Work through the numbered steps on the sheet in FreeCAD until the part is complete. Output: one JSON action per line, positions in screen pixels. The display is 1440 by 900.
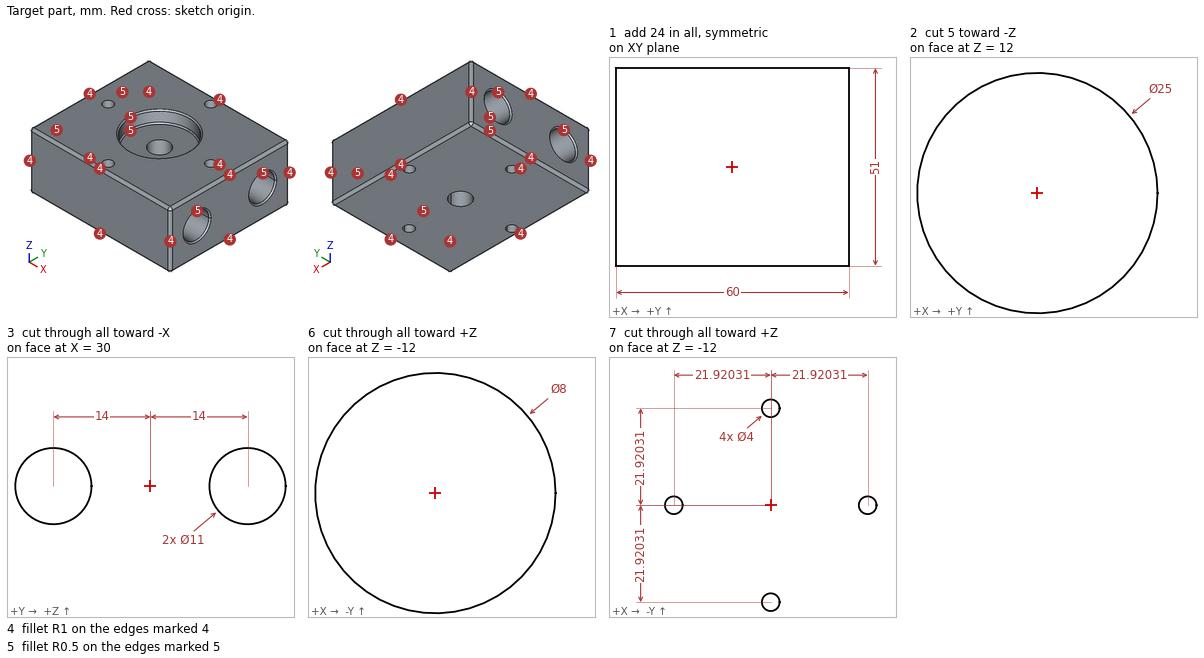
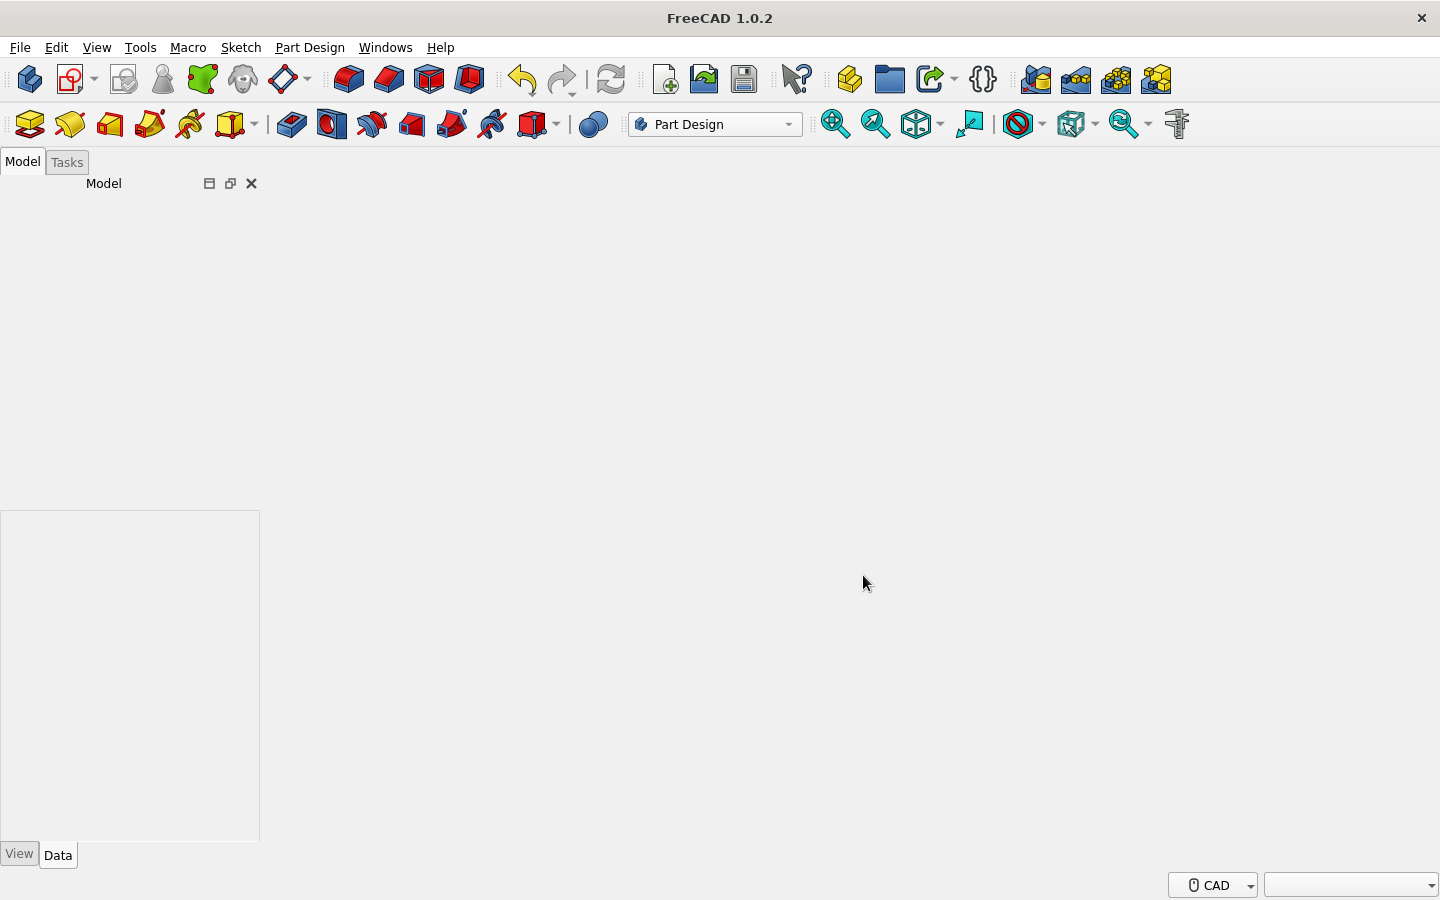
{"action": "left_click", "coordinate": [664, 80]}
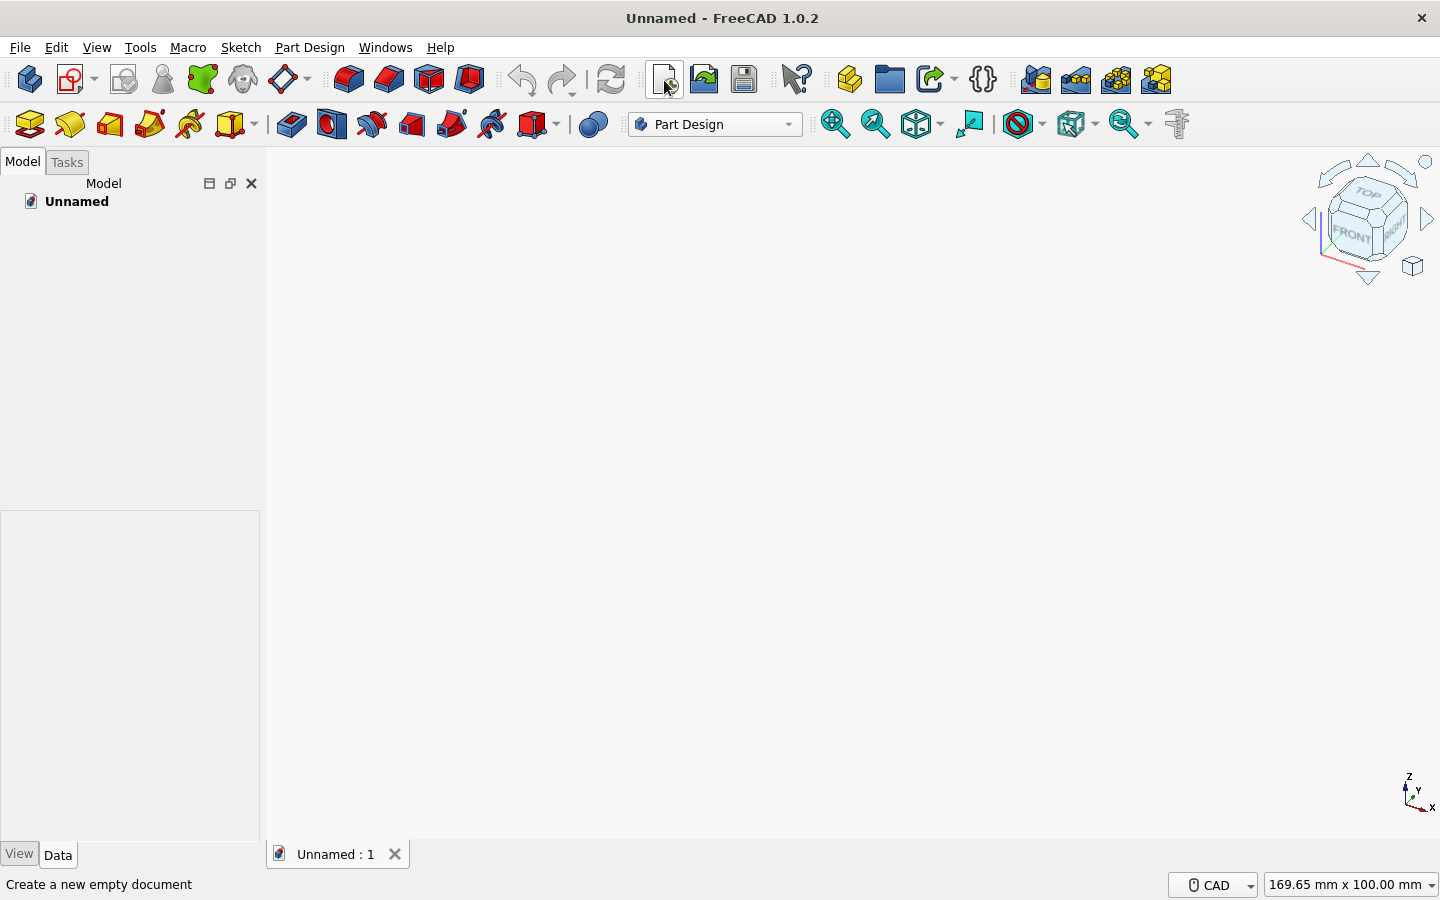
{"action": "left_click", "coordinate": [70, 80]}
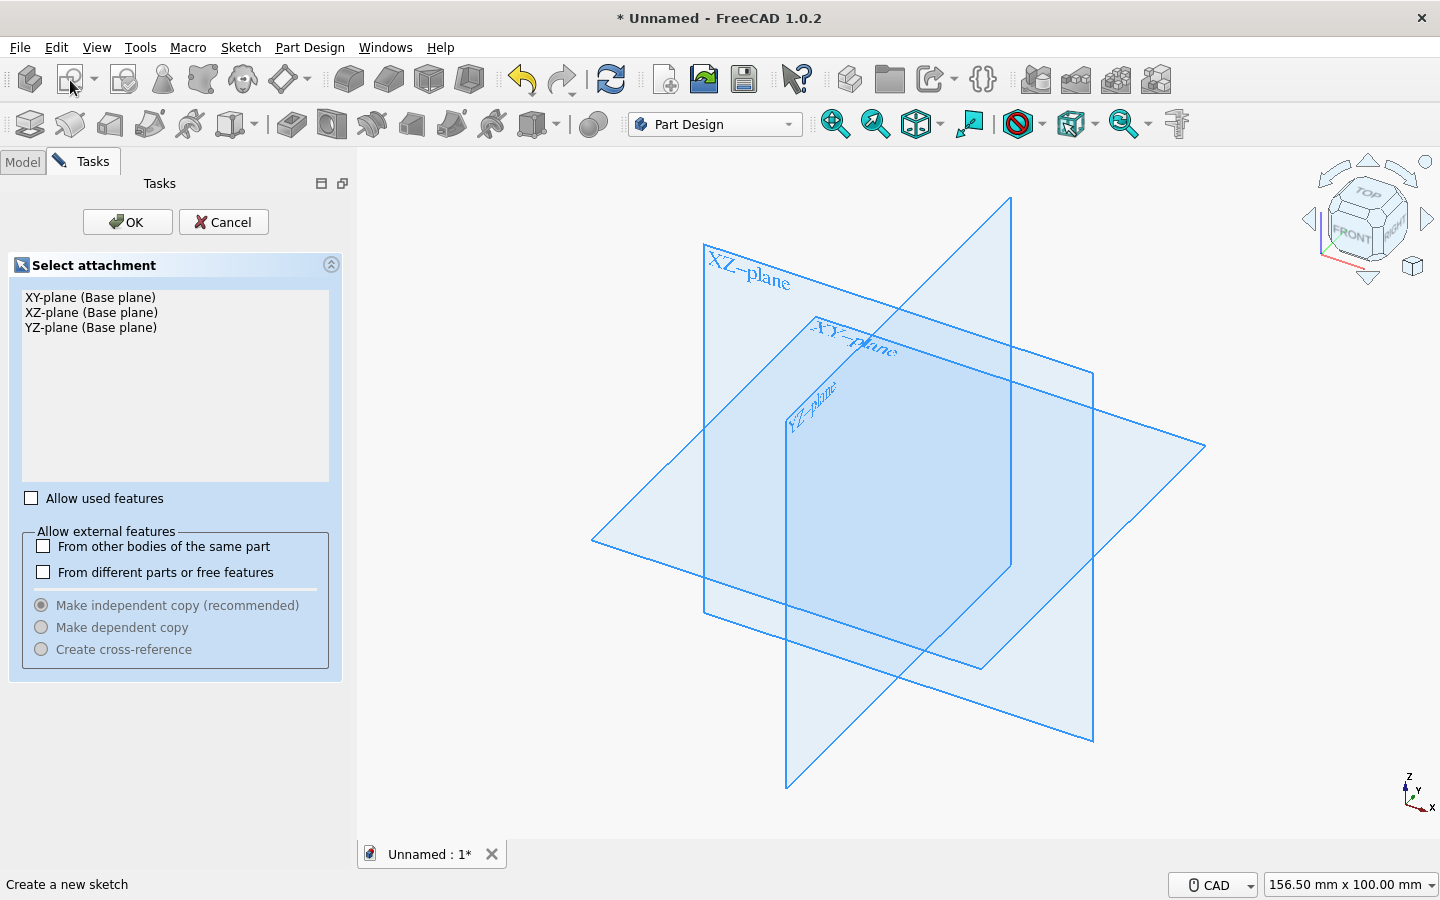
{"action": "left_click", "coordinate": [82, 298]}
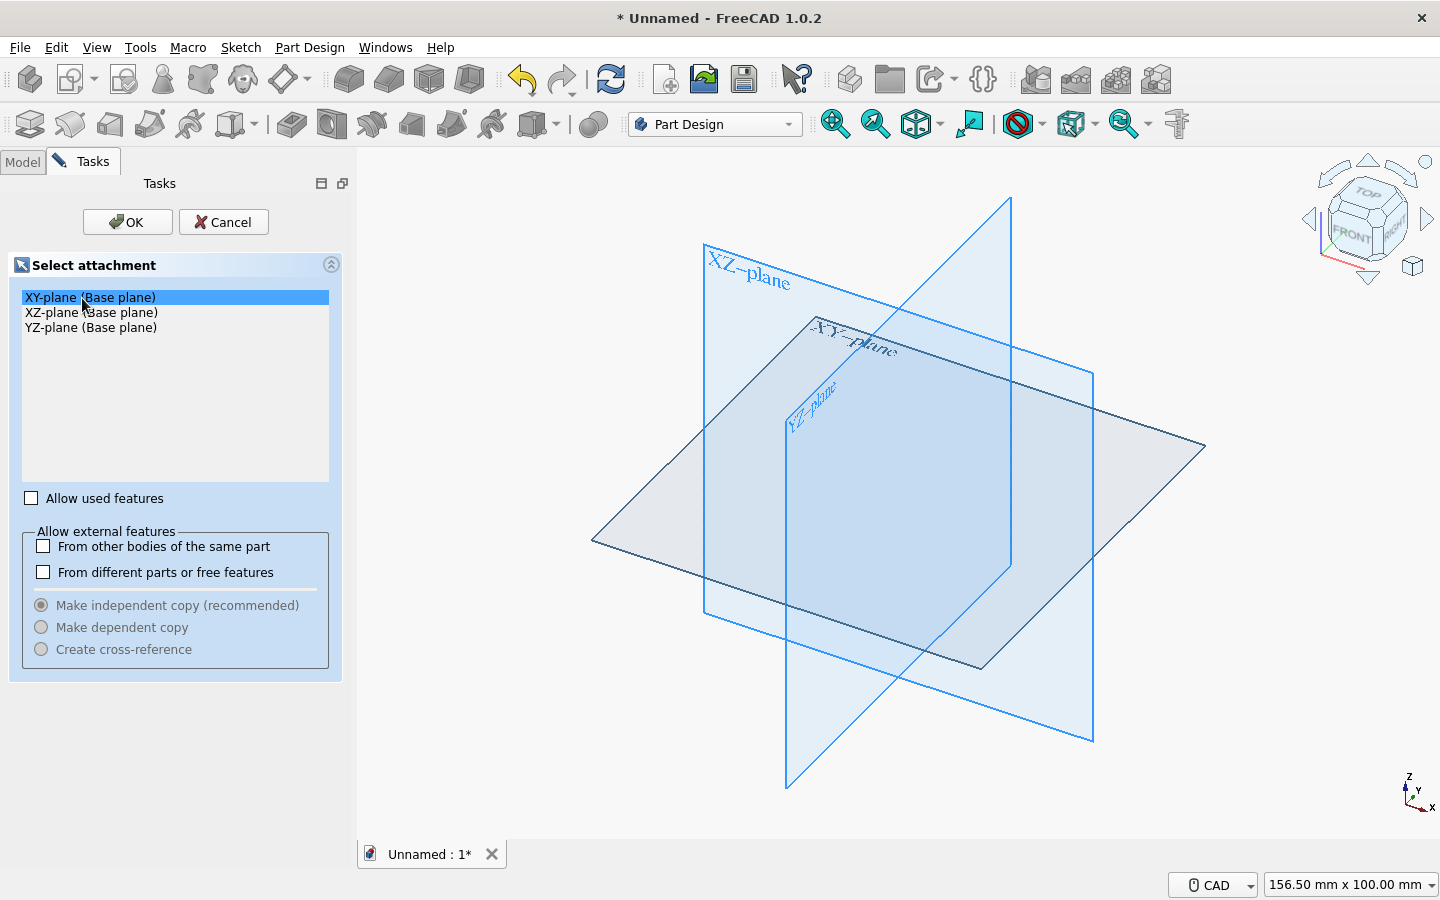
{"action": "left_click", "coordinate": [128, 222]}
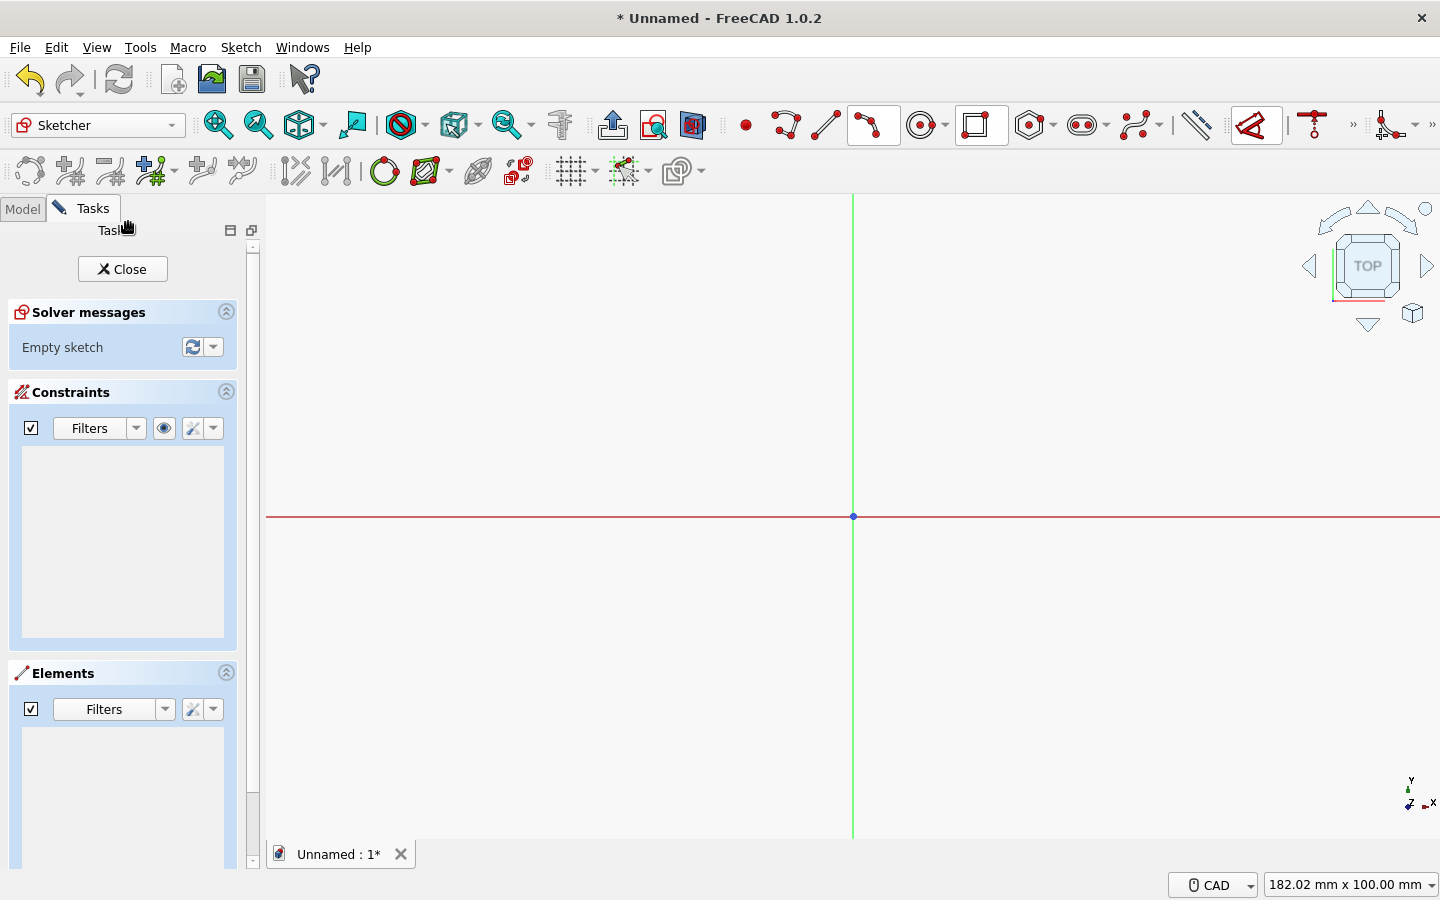
{"action": "left_click", "coordinate": [1002, 126]}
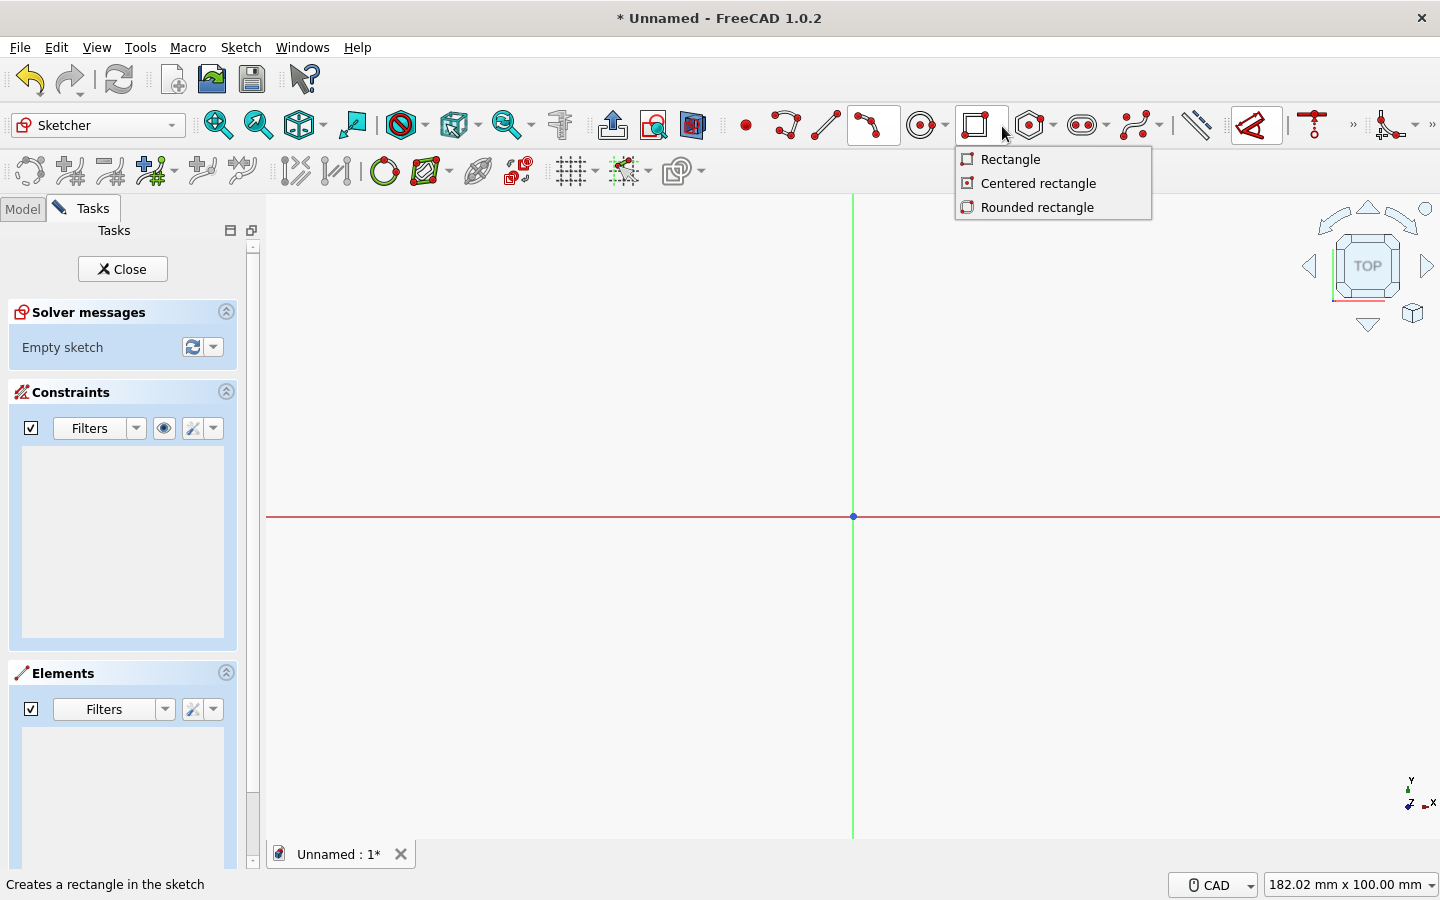
{"action": "left_click", "coordinate": [1054, 183]}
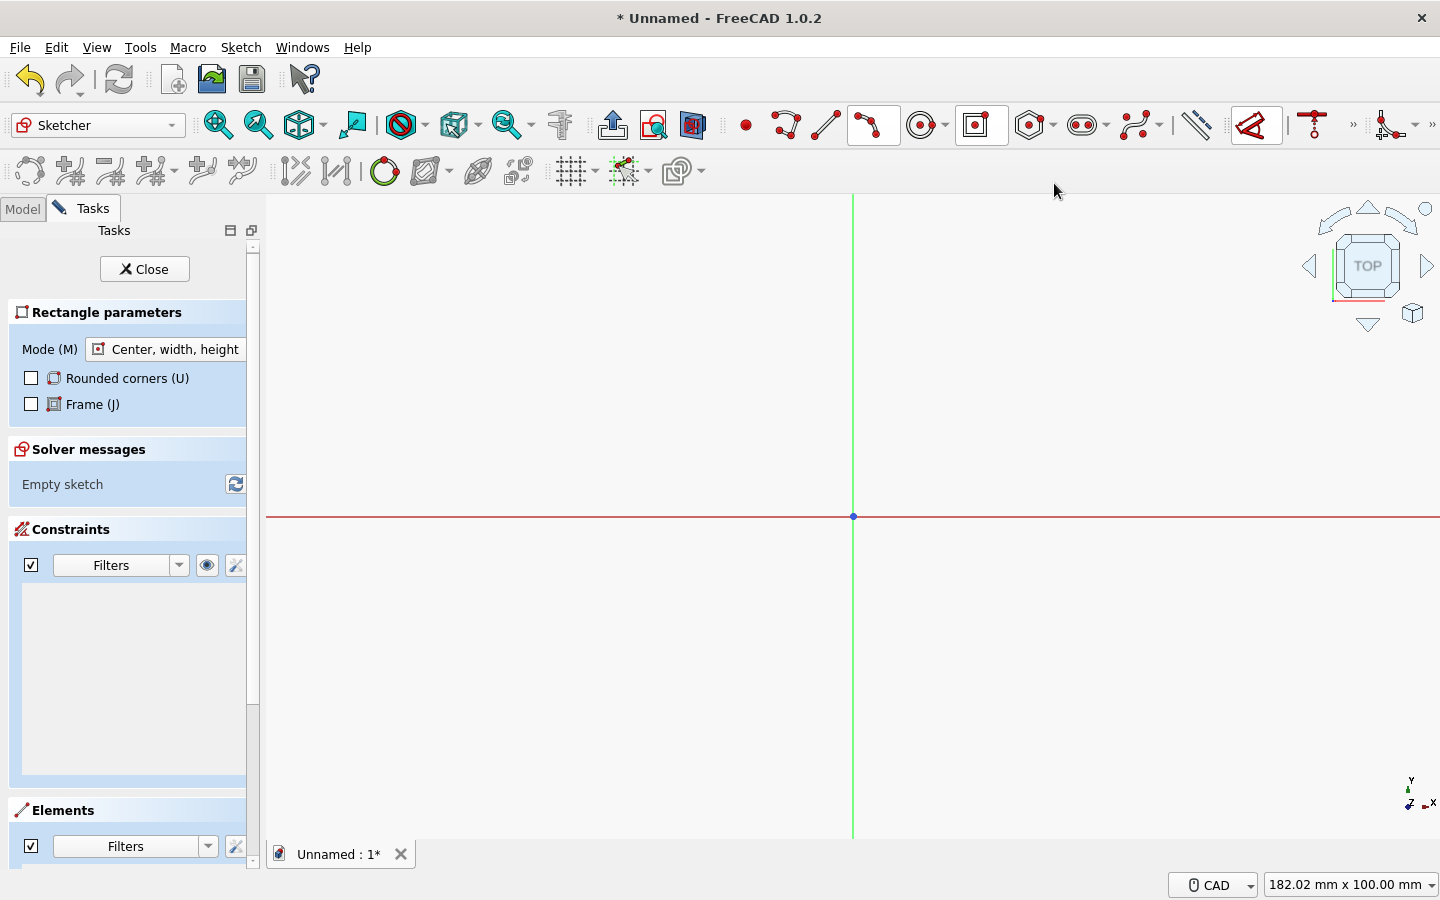
{"action": "left_click", "coordinate": [853, 516]}
{"action": "left_click", "coordinate": [1046, 352]}
{"action": "key", "text": "Escape"}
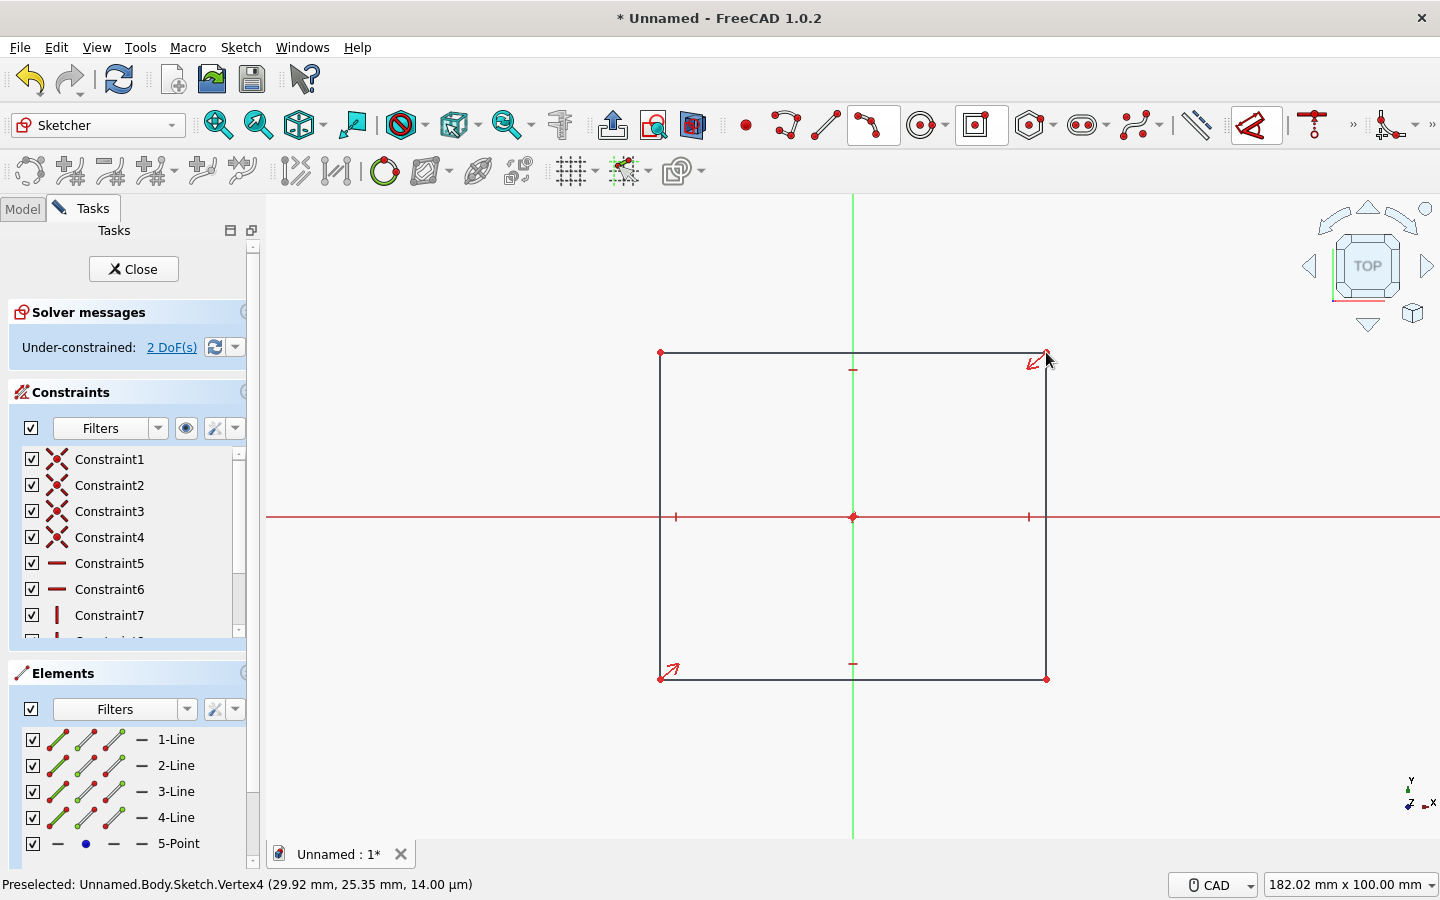
{"action": "key", "text": "d"}